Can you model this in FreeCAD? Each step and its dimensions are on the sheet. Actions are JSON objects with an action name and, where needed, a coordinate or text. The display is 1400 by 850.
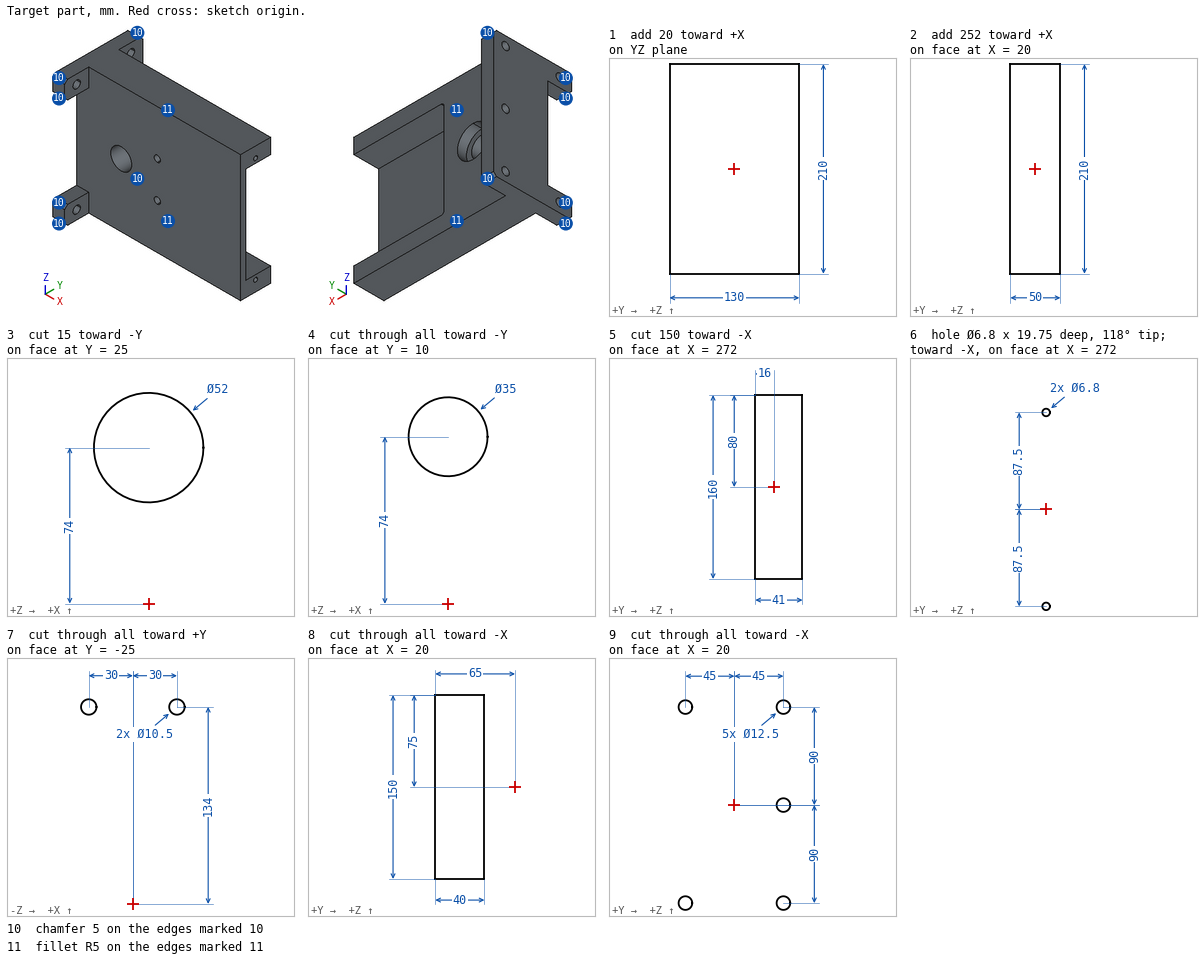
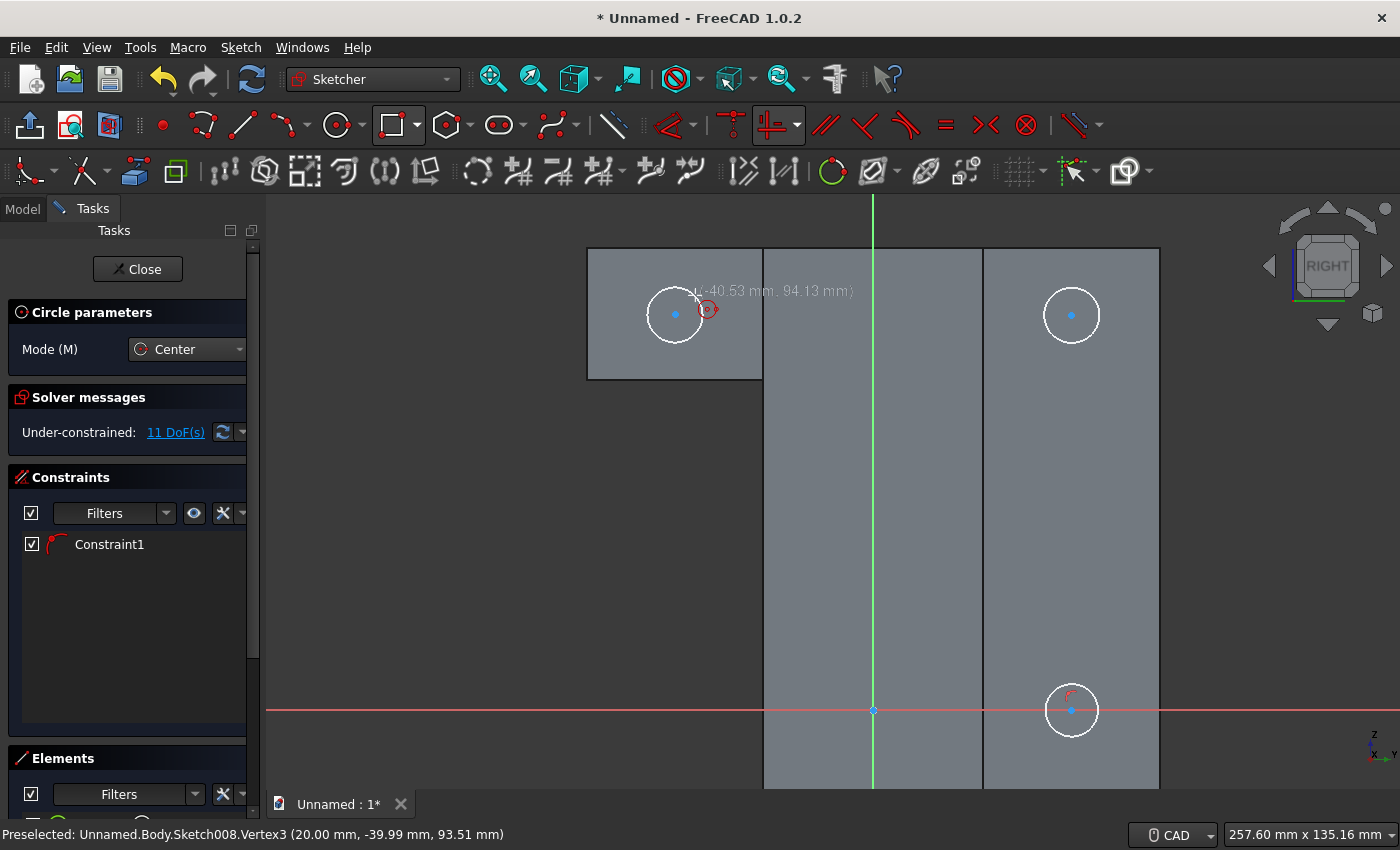
{"action": "scroll", "coordinate": [676, 313], "scroll_direction": "down", "scroll_amount": 4}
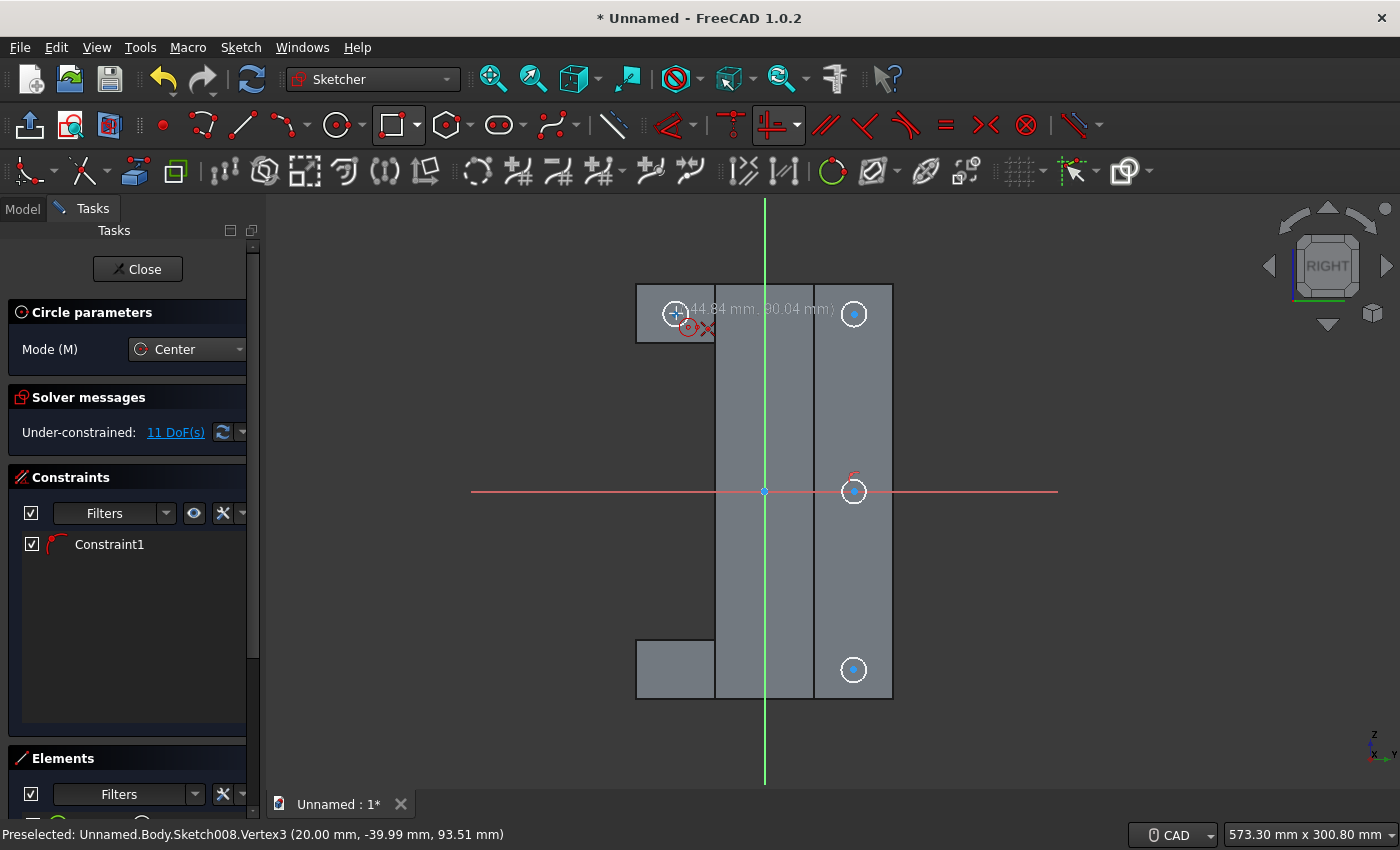
{"action": "scroll", "coordinate": [676, 670], "scroll_direction": "up", "scroll_amount": 4}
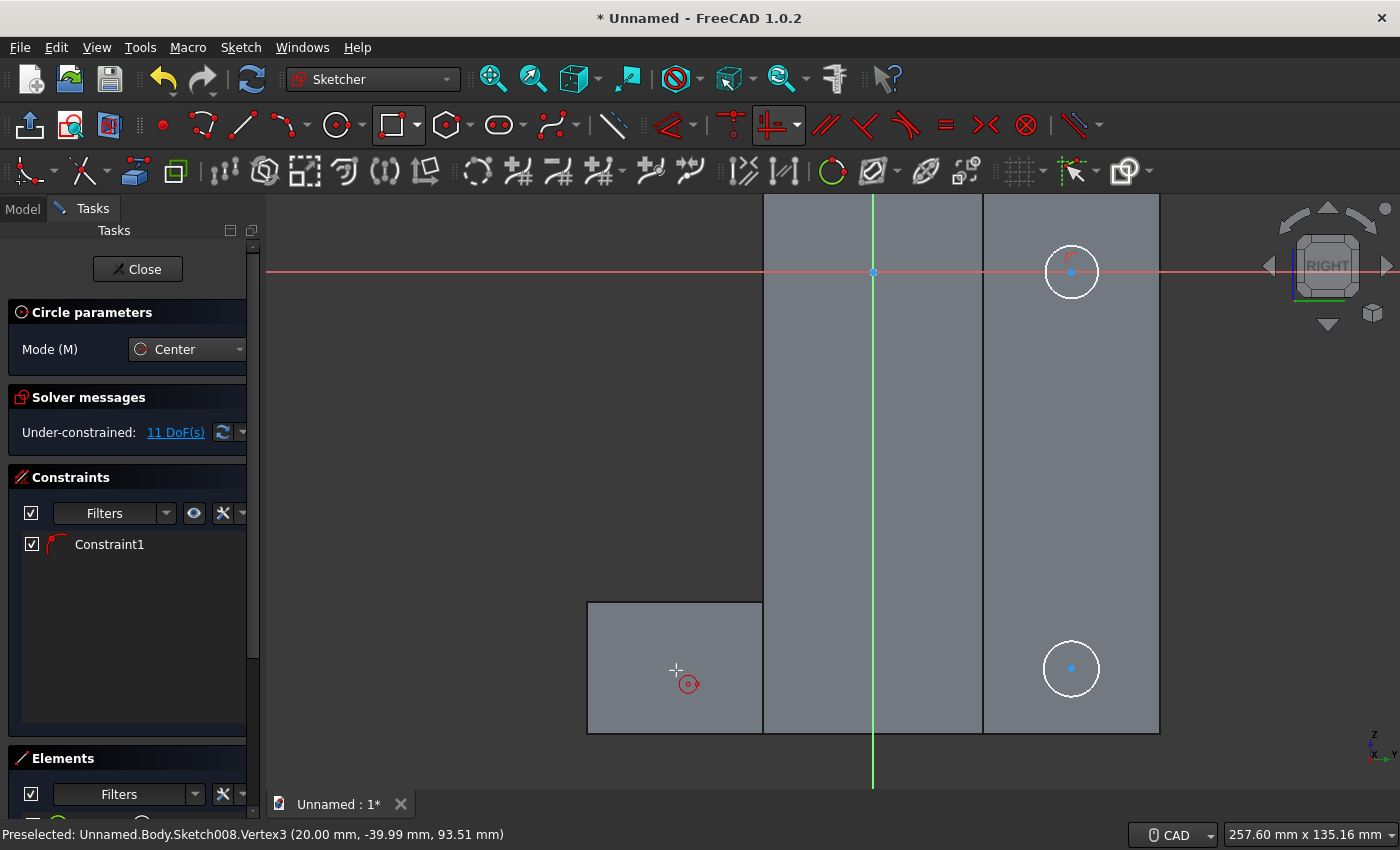
{"action": "left_click", "coordinate": [675, 668]}
{"action": "left_click", "coordinate": [695, 649]}
{"action": "key", "text": "Escape"}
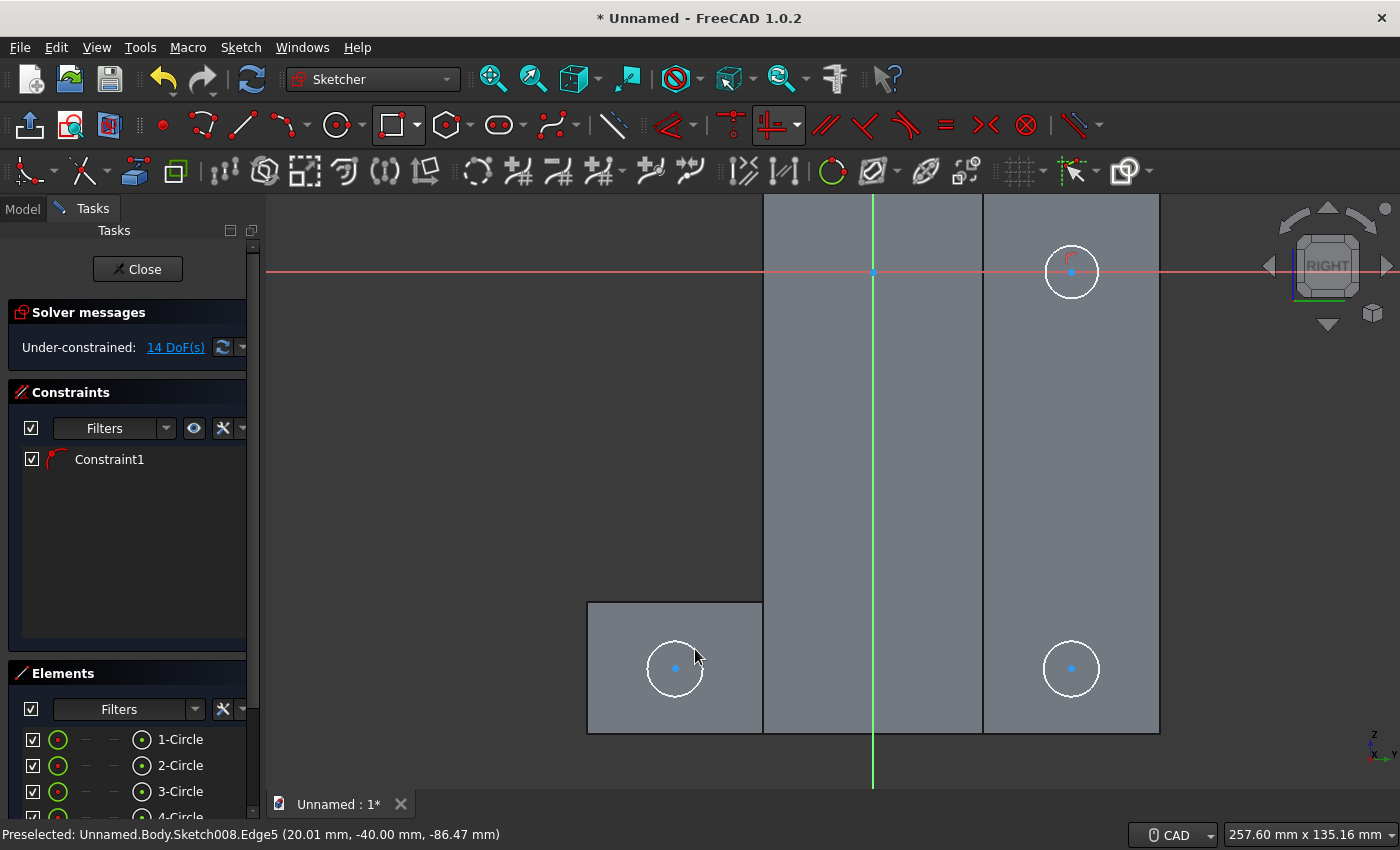
{"action": "scroll", "coordinate": [676, 671], "scroll_direction": "down", "scroll_amount": 4}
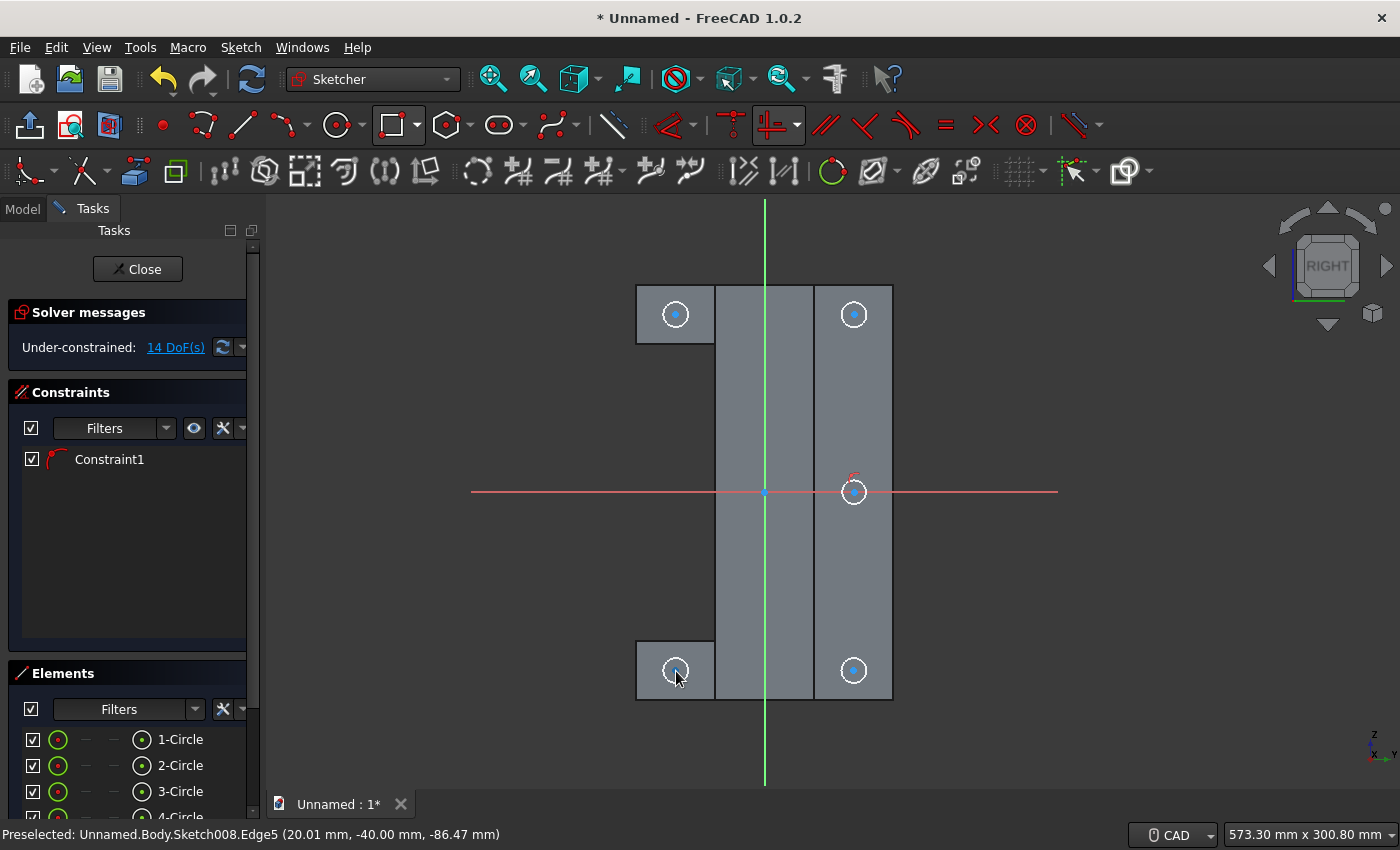
{"action": "left_click", "coordinate": [863, 306]}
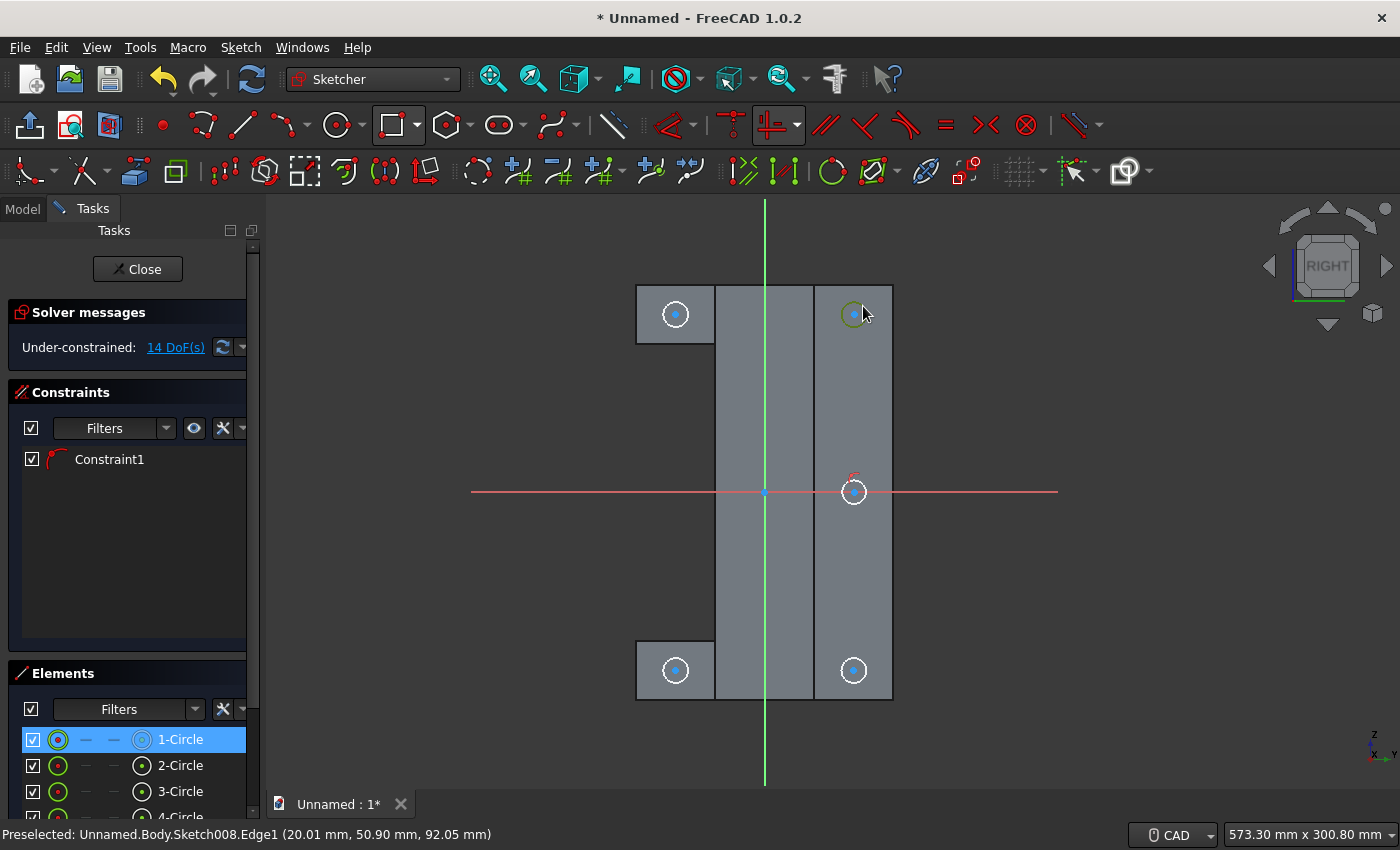
{"action": "left_click", "coordinate": [842, 492]}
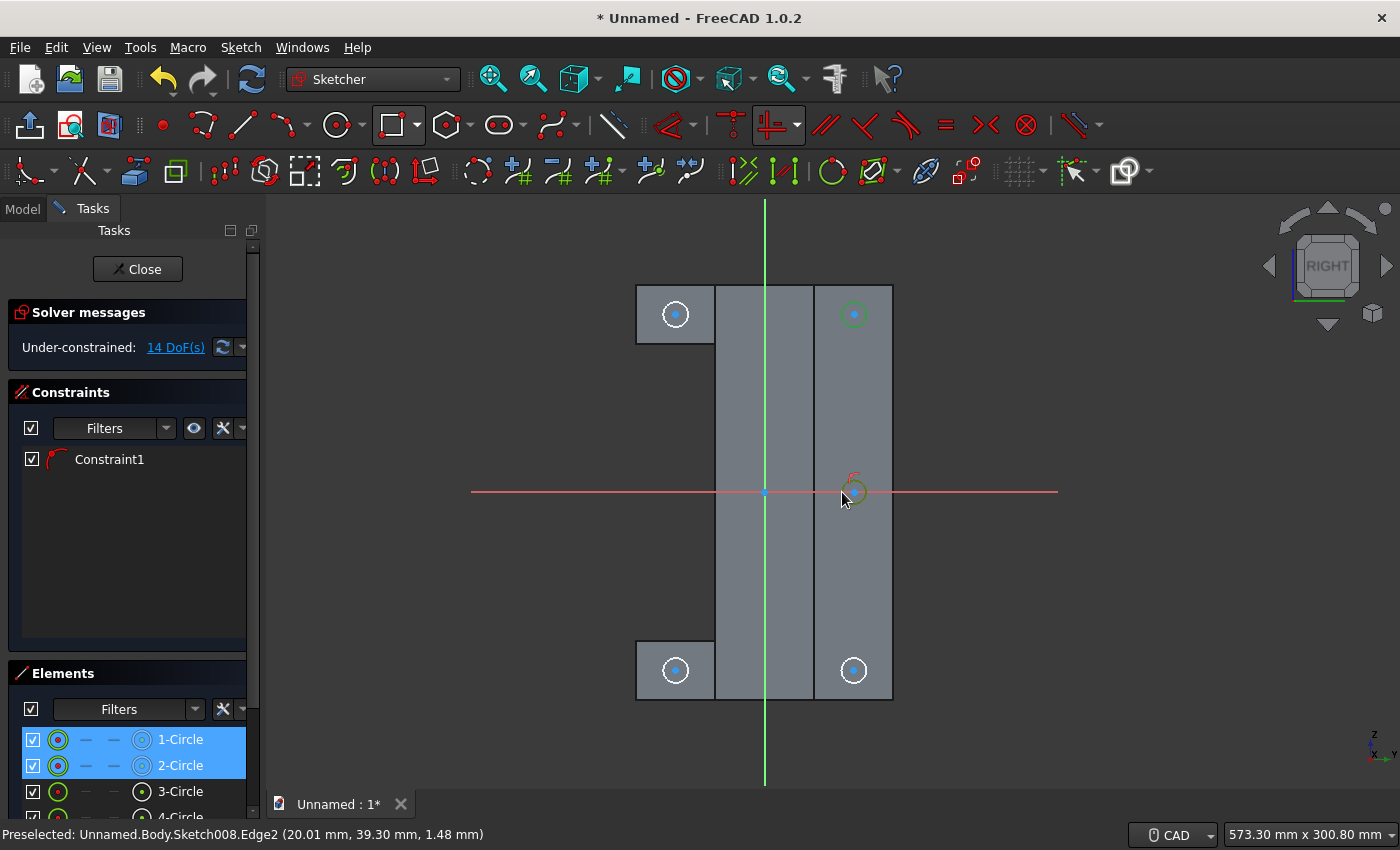
{"action": "left_click", "coordinate": [863, 662]}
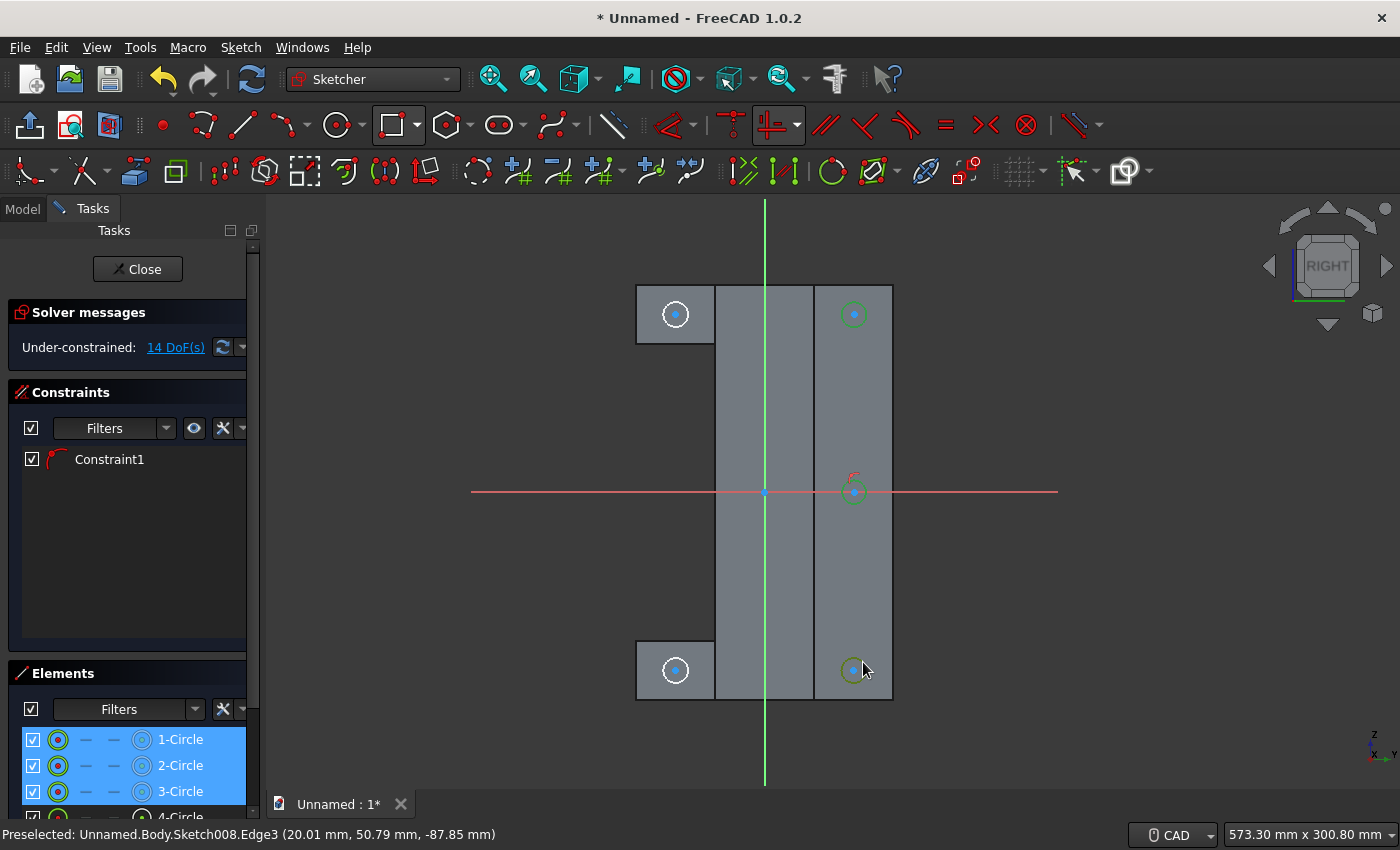
{"action": "left_click", "coordinate": [684, 306]}